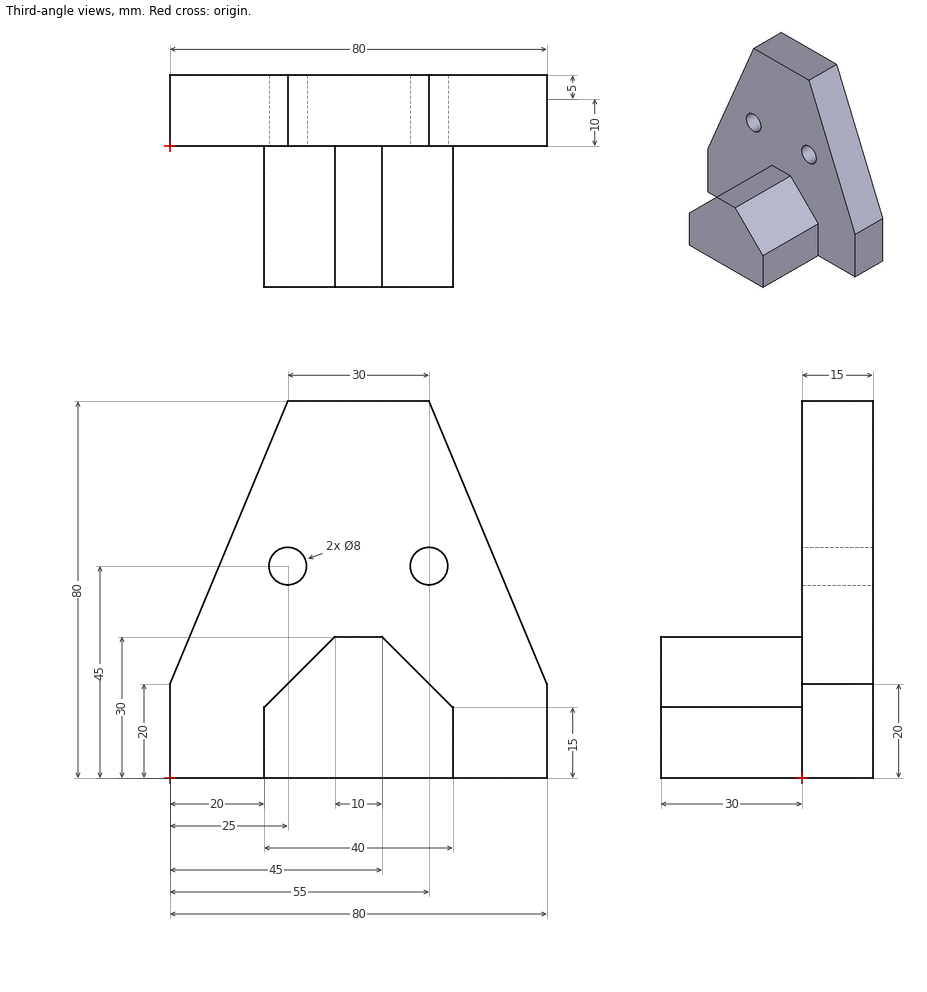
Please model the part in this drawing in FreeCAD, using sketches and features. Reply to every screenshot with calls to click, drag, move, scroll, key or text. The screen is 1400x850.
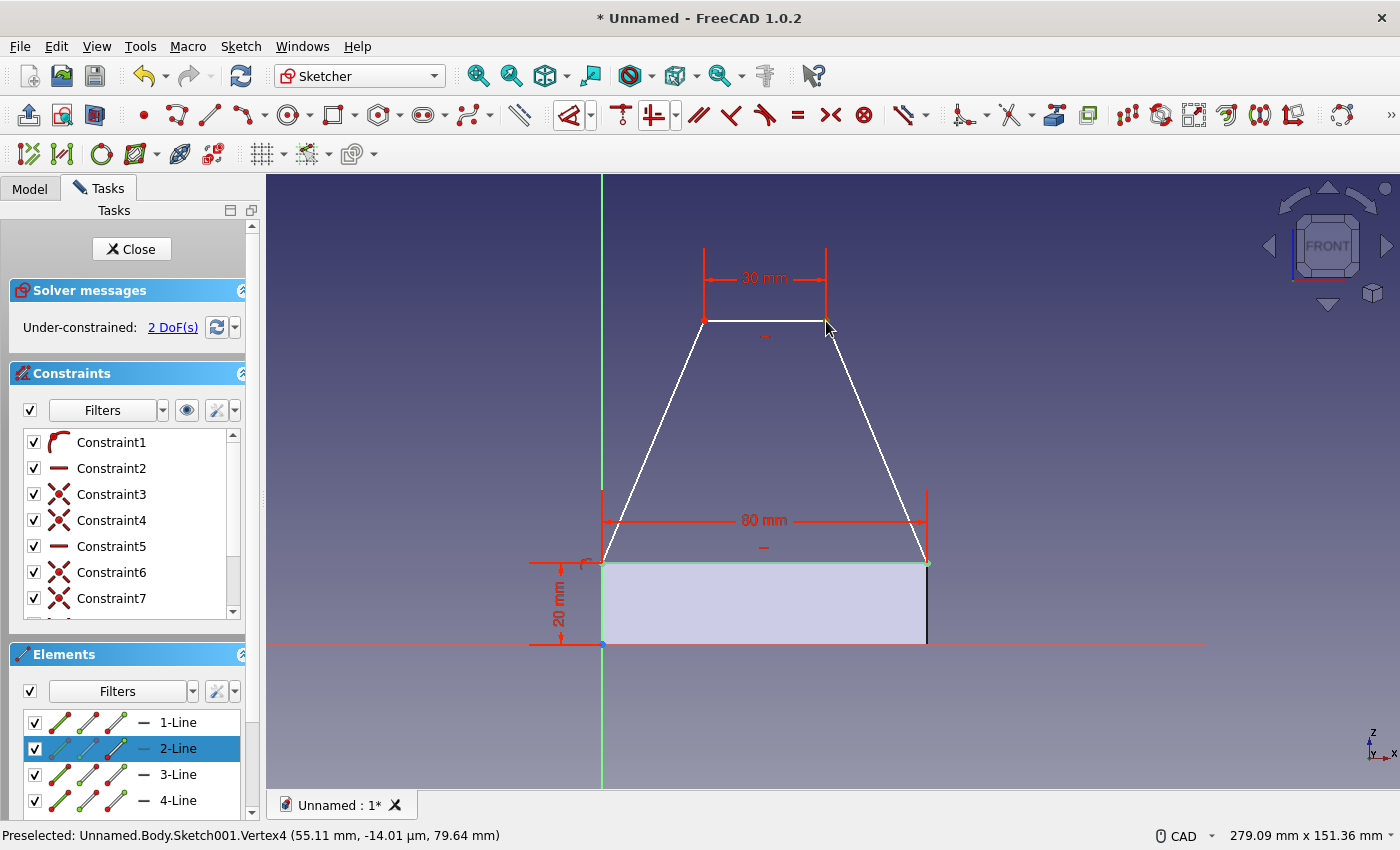
key(l)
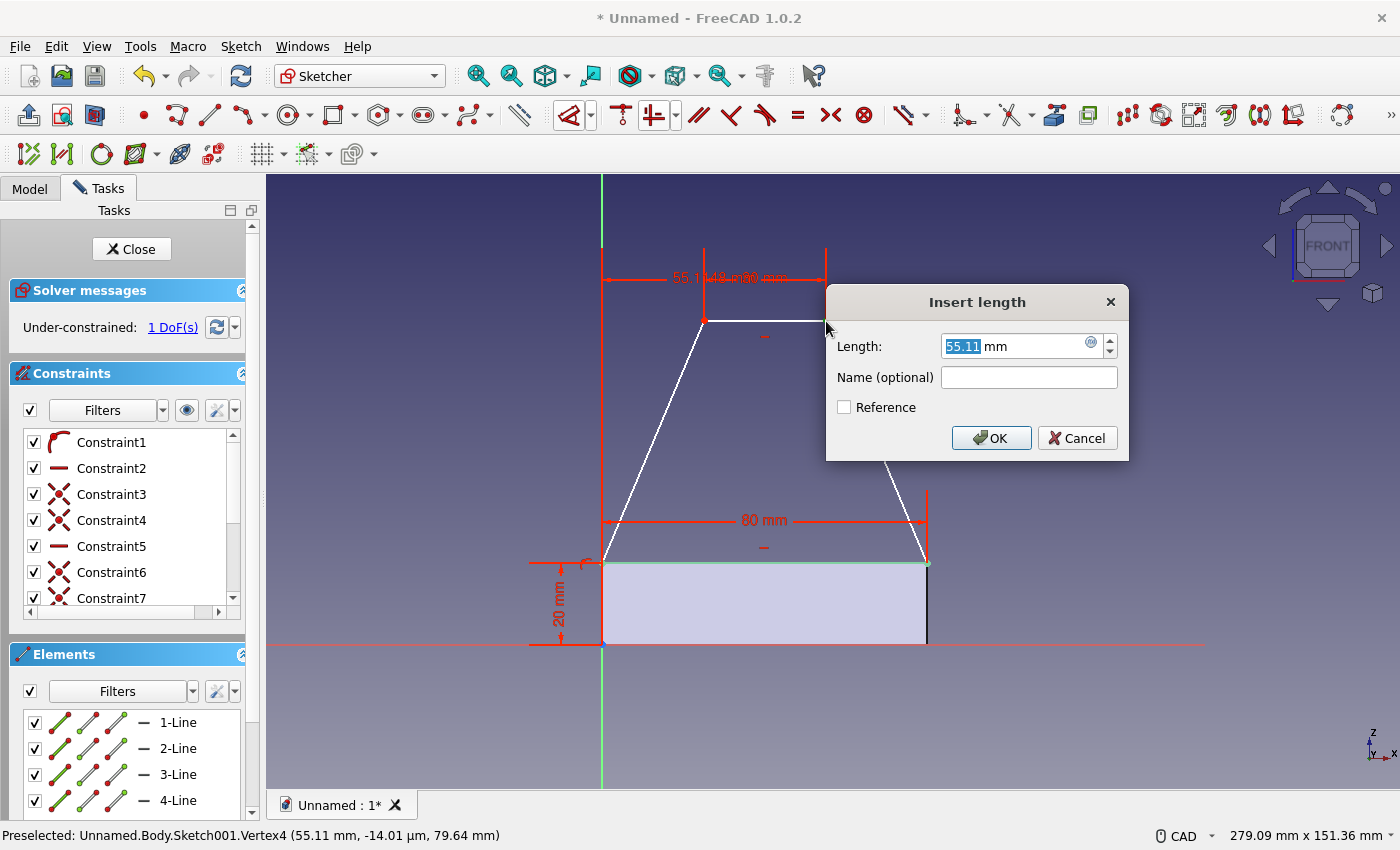
text(55)
key(Return)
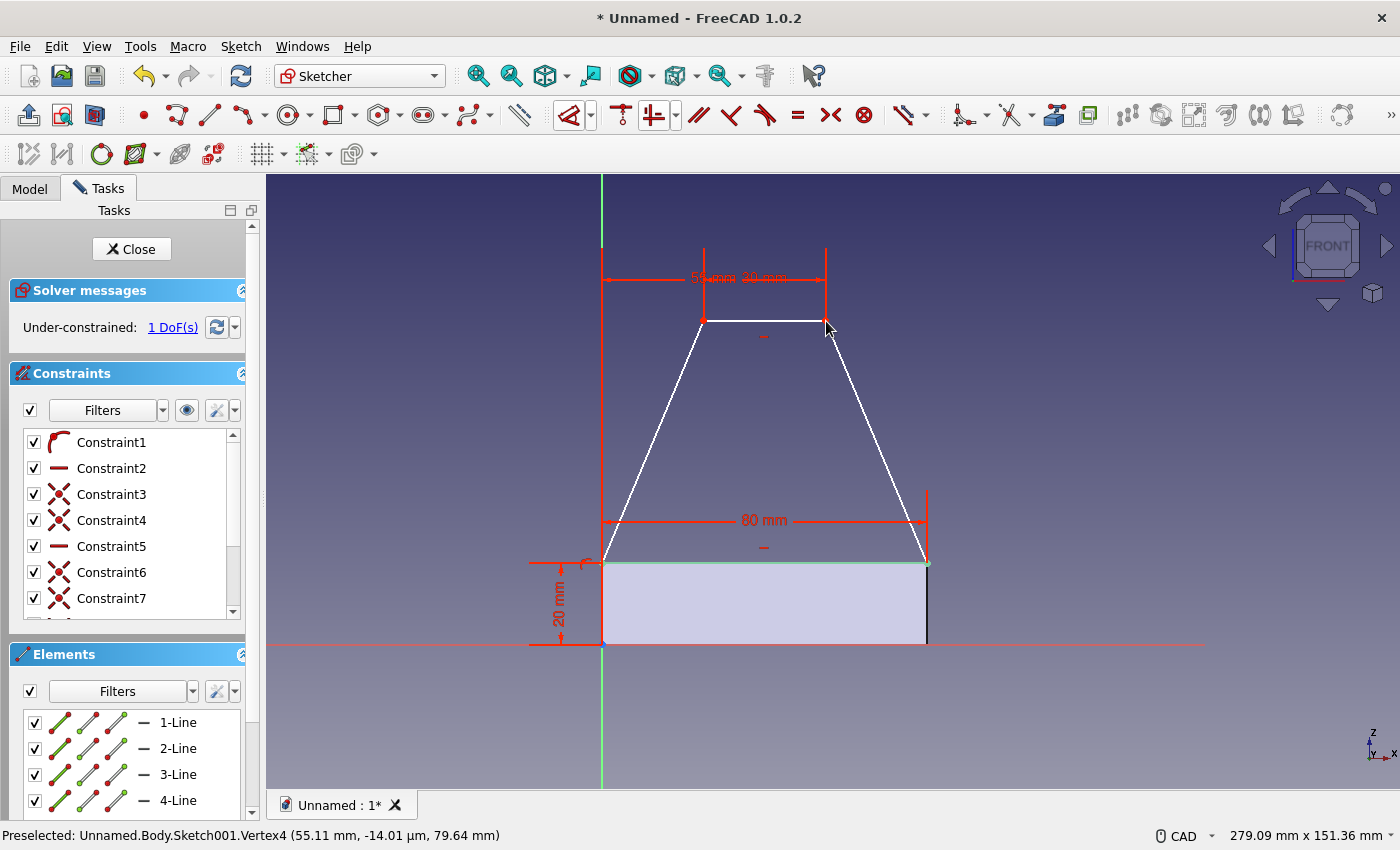
click(826, 321)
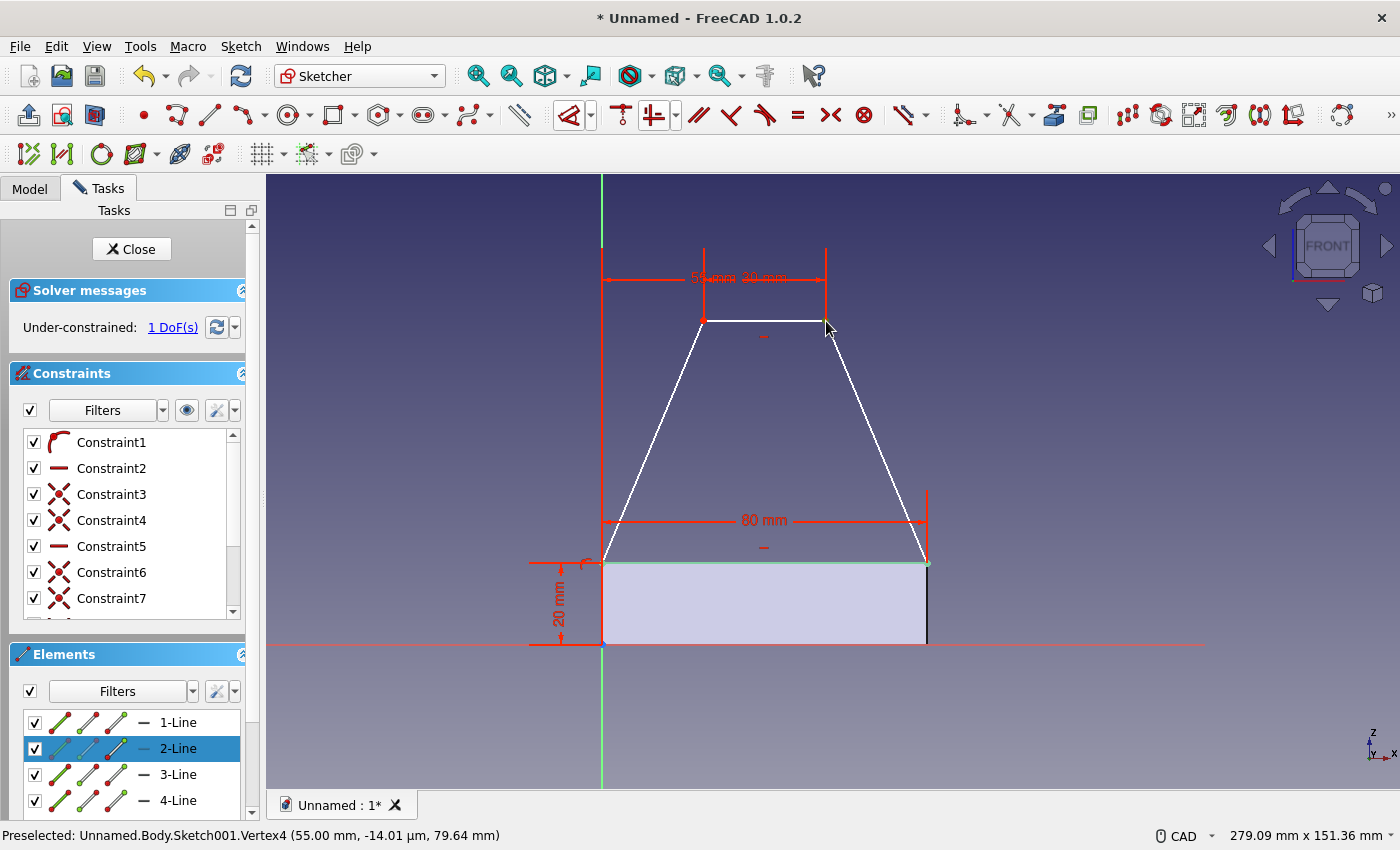
key(i)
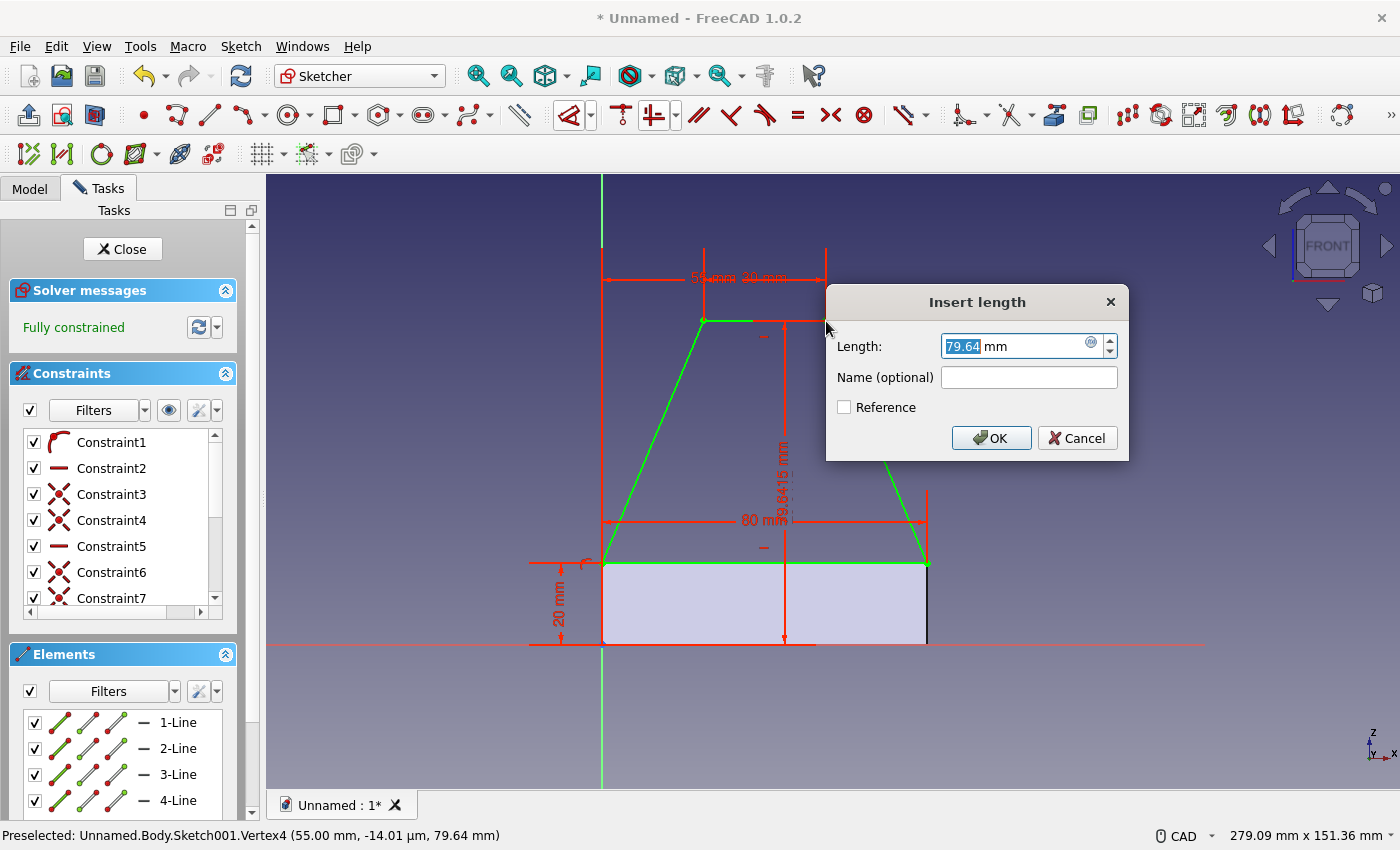
text(80)
key(Return)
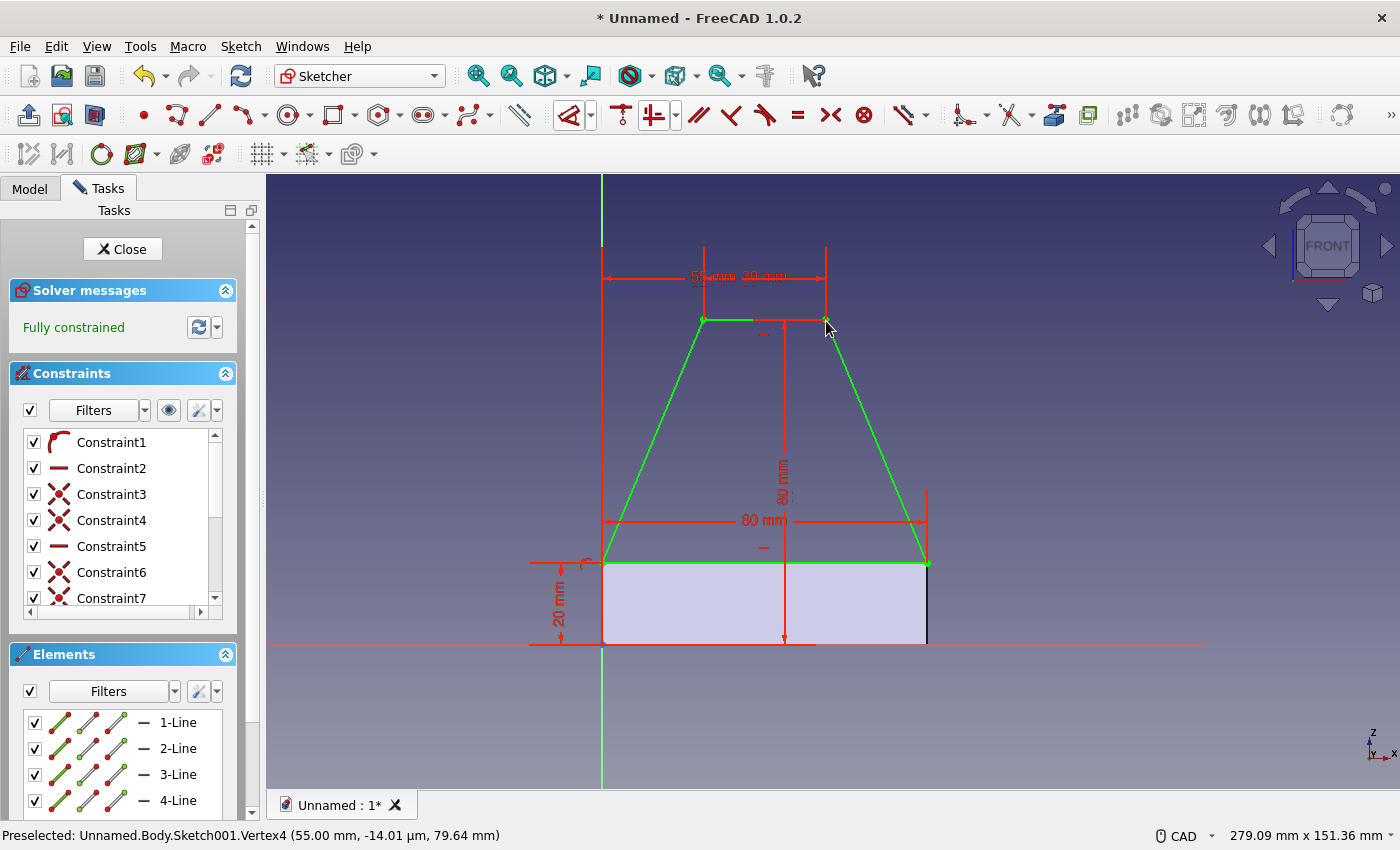
click(123, 249)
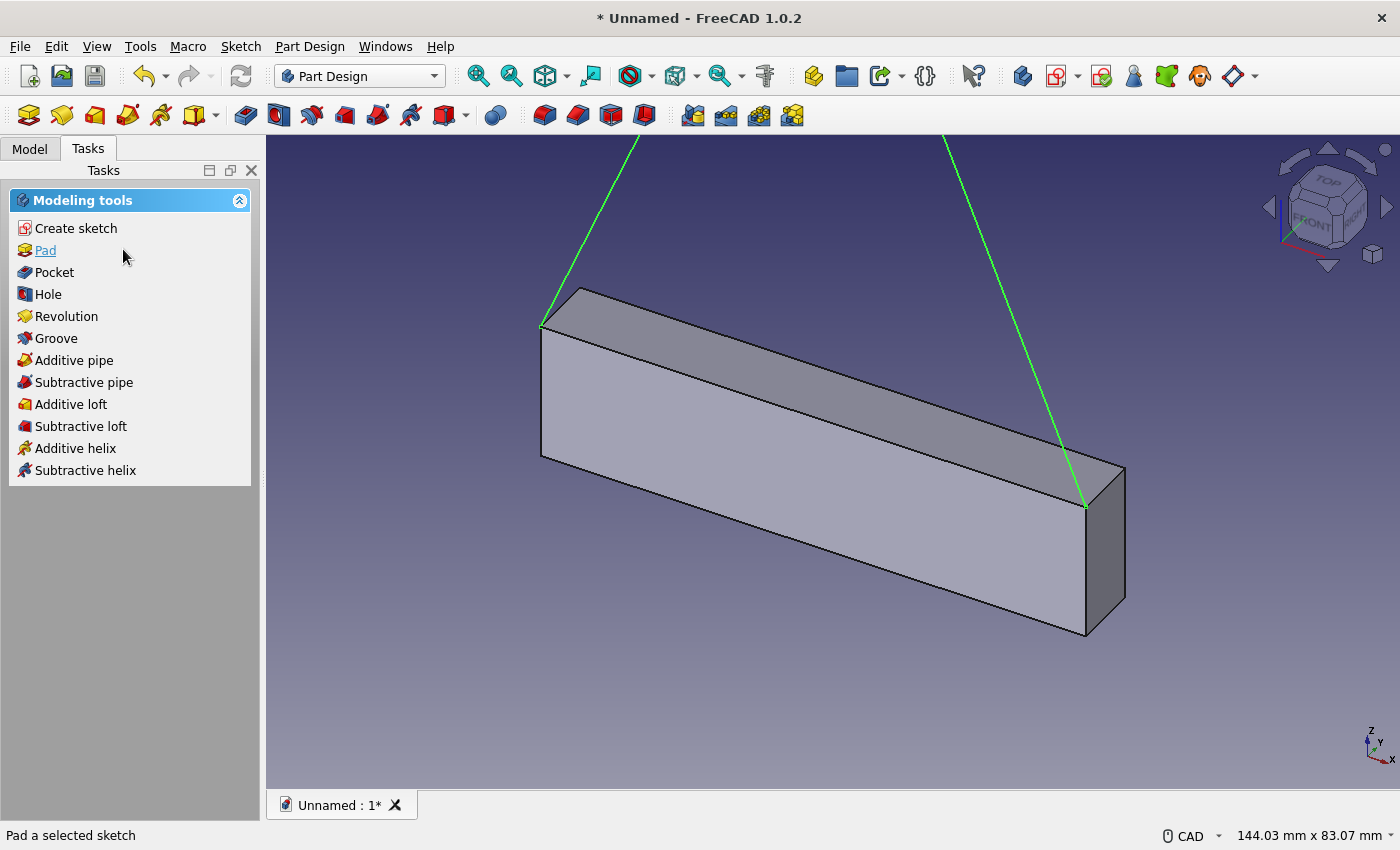
click(29, 116)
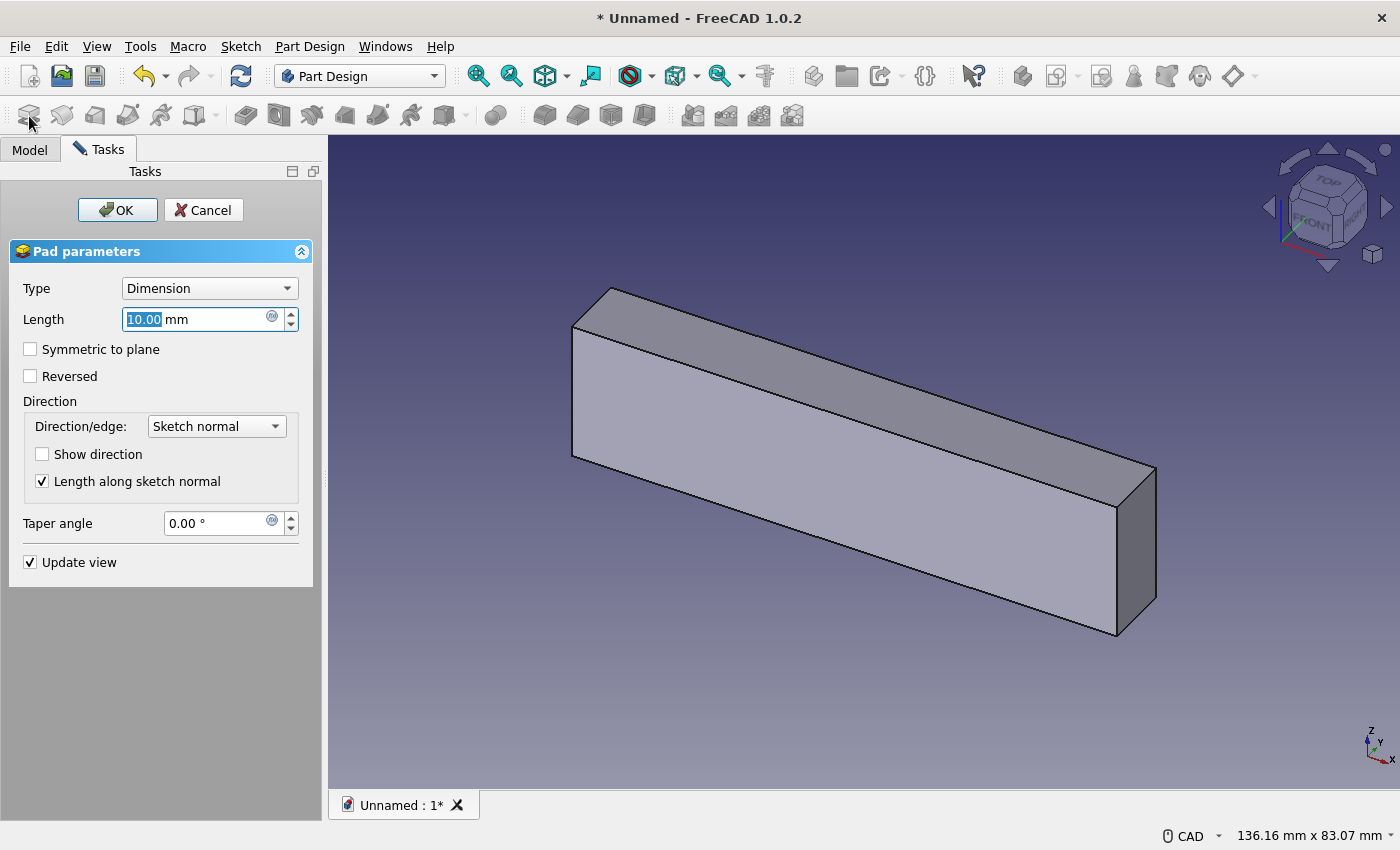
text(15)
key(Tab)